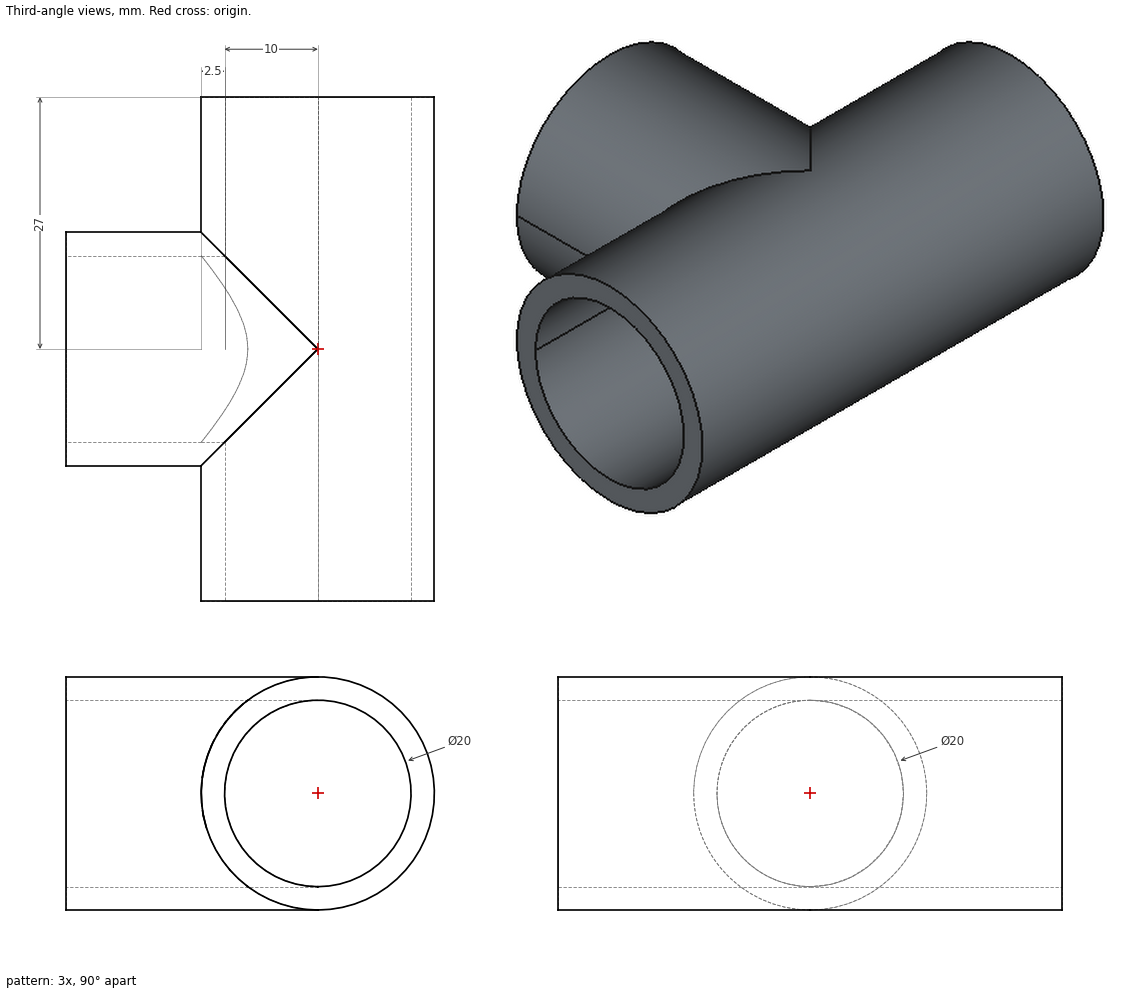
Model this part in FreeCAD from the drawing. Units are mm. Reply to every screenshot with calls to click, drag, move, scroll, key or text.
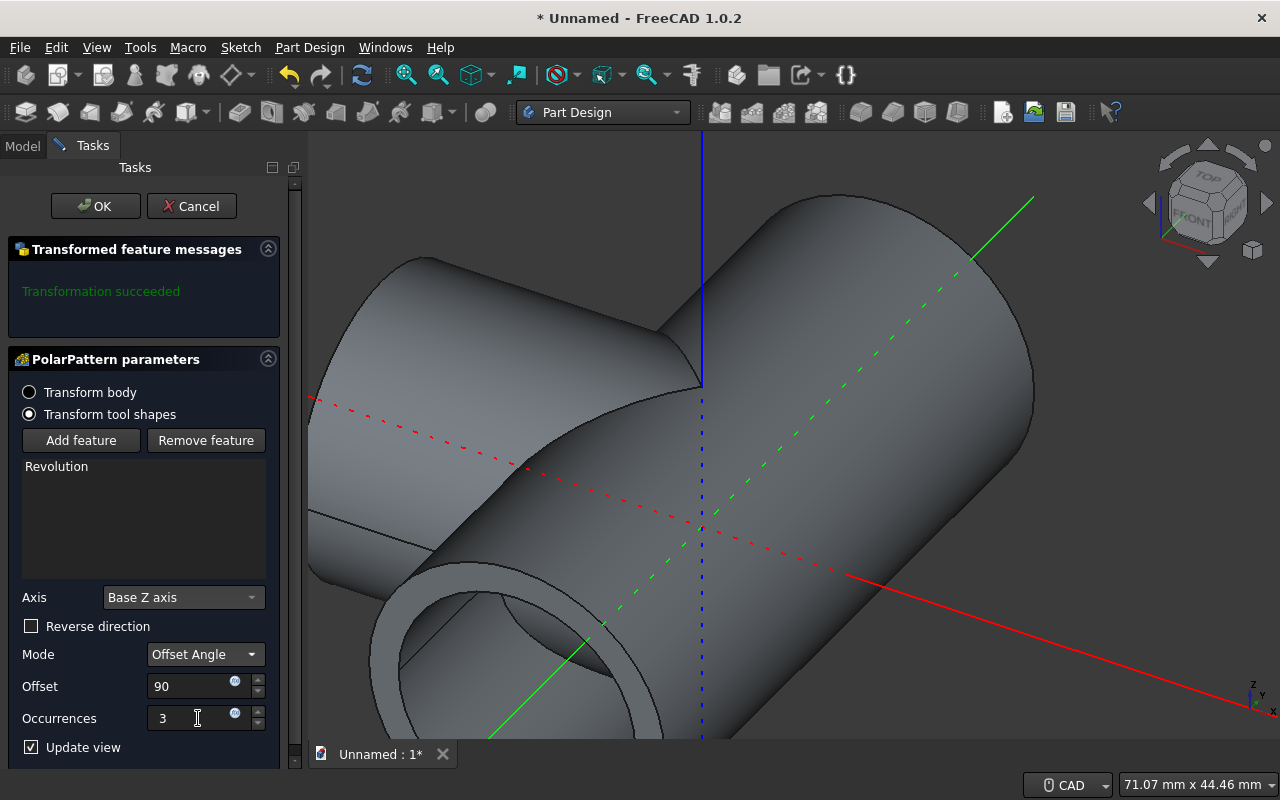
click(96, 206)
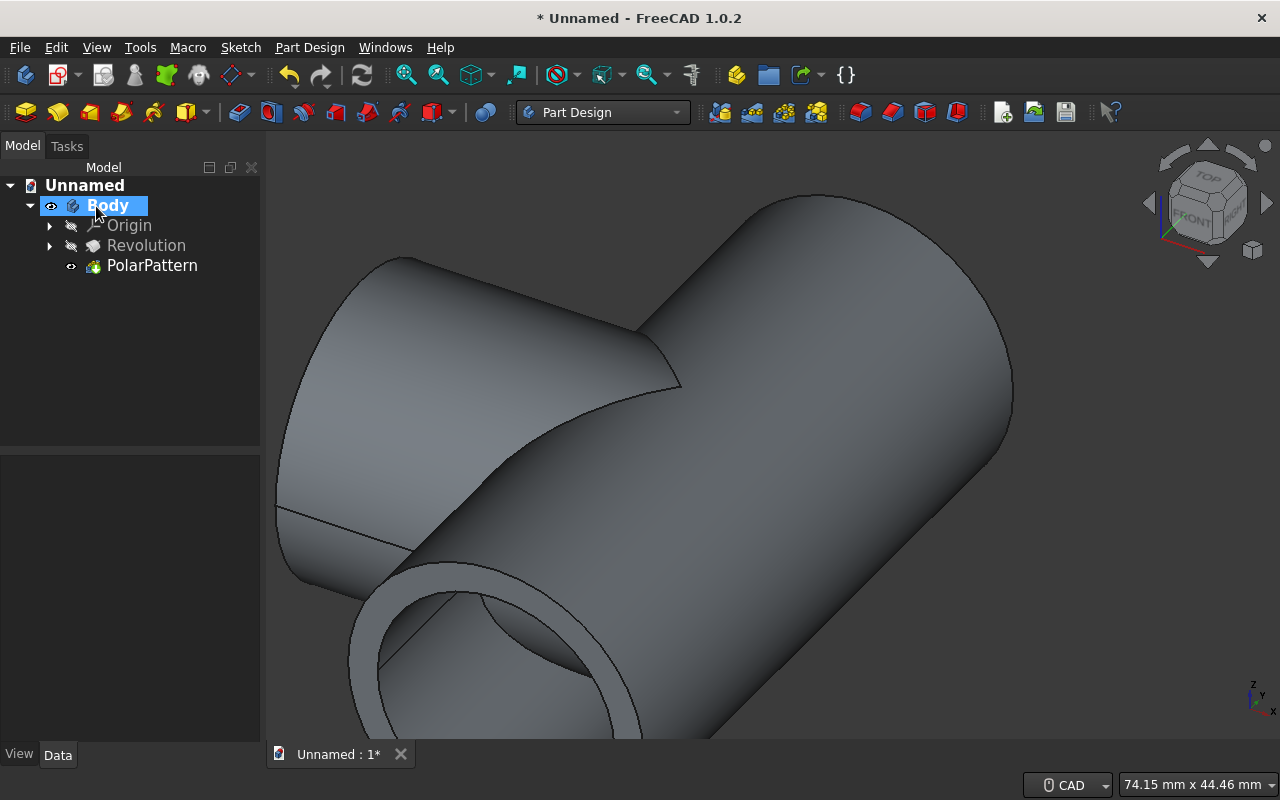
key(v)
key(f)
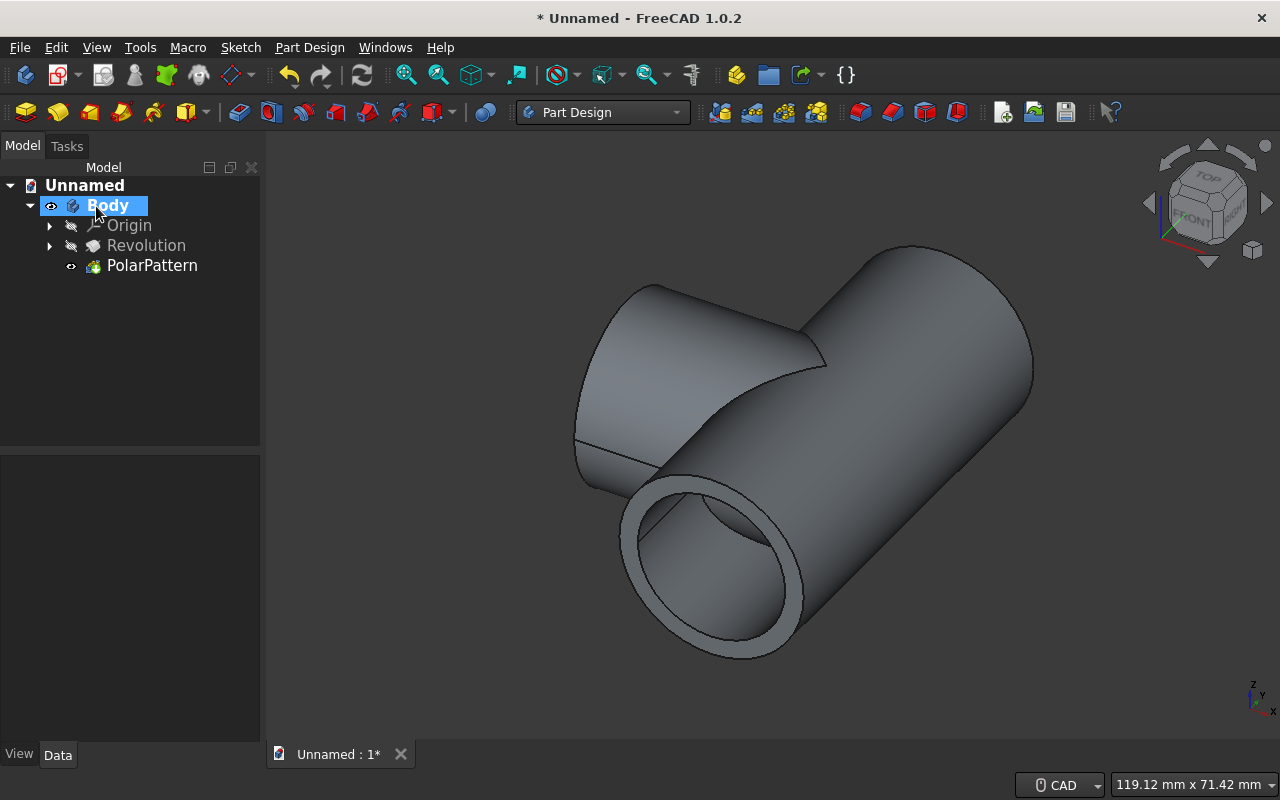
click(738, 649)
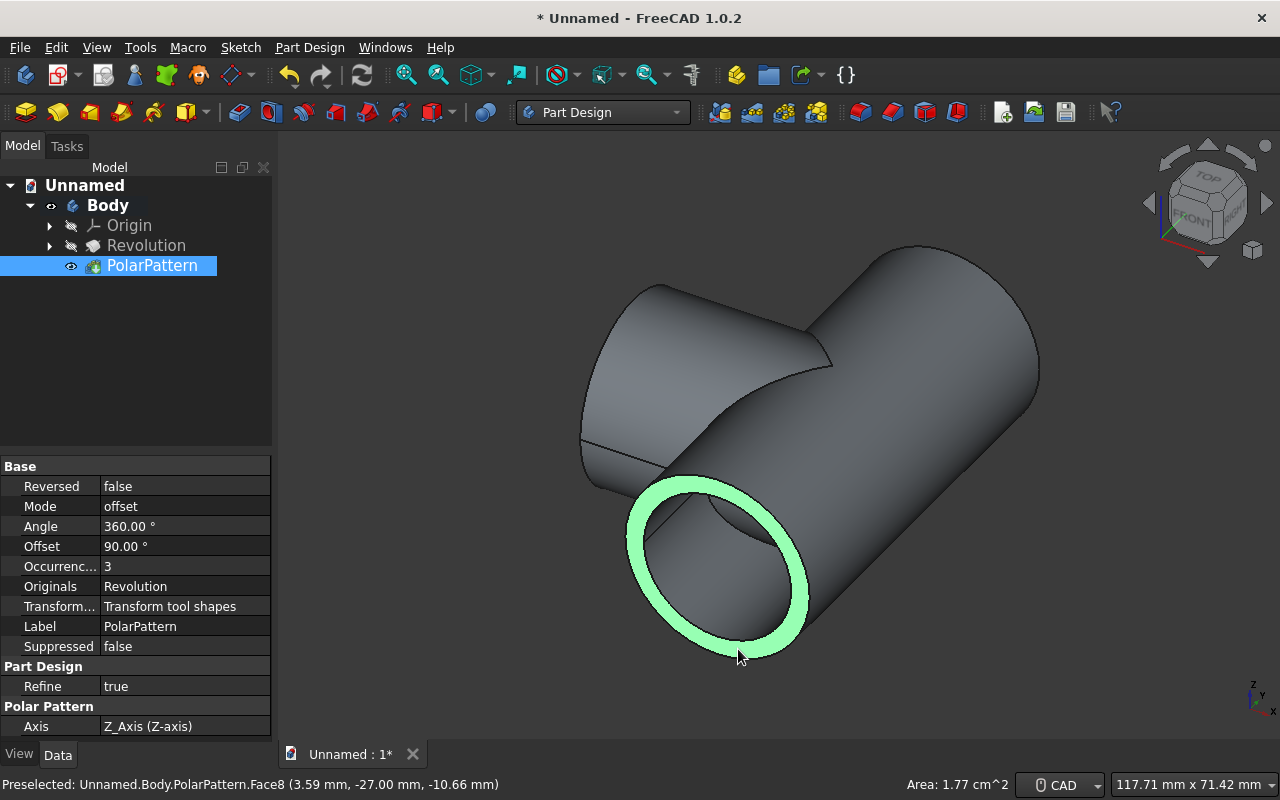
click(58, 76)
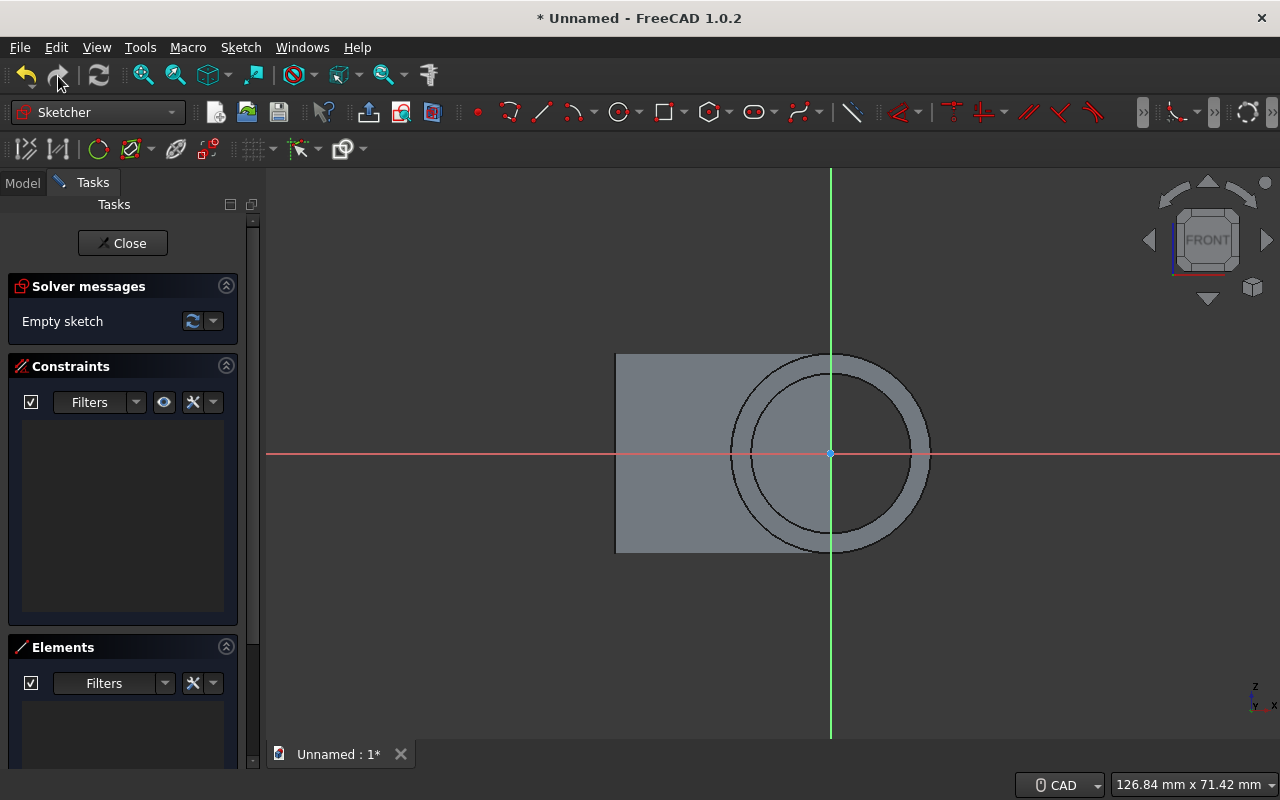
scroll(934, 454, up, 4)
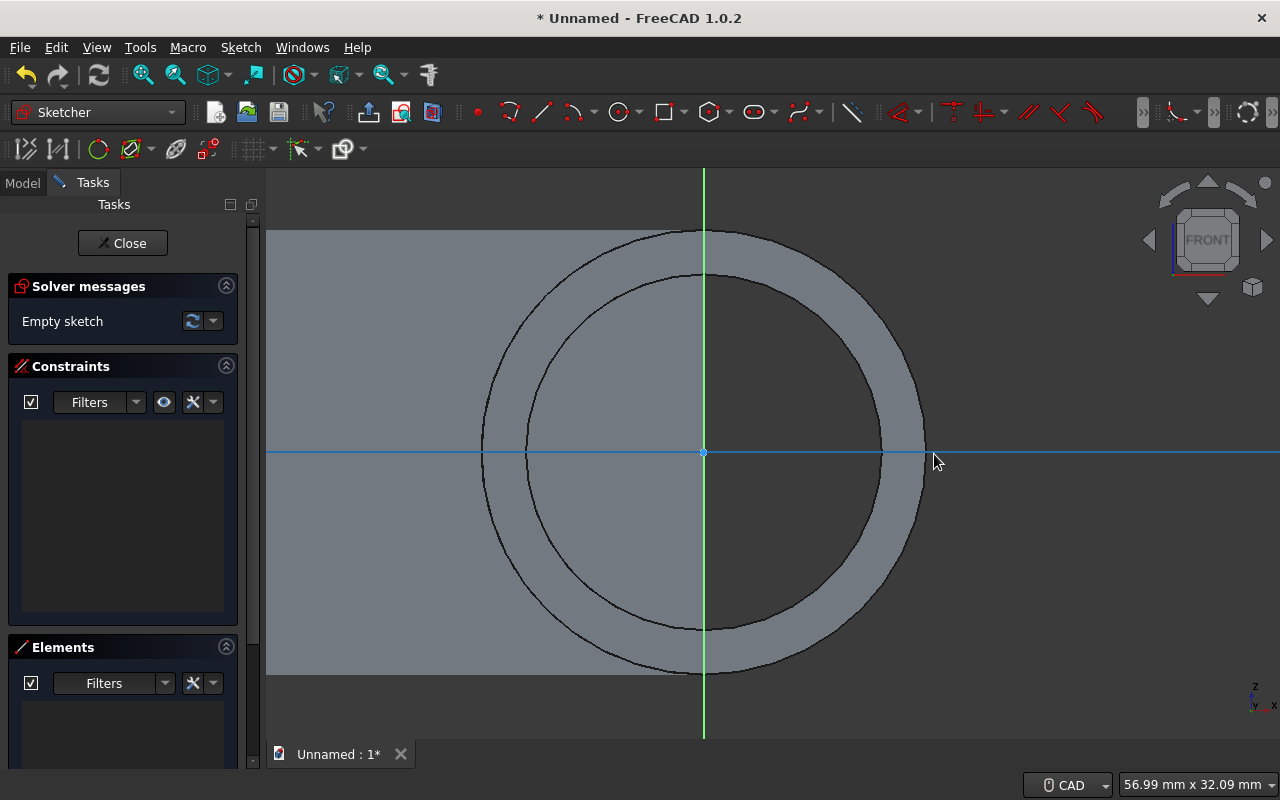
key(g)
key(c)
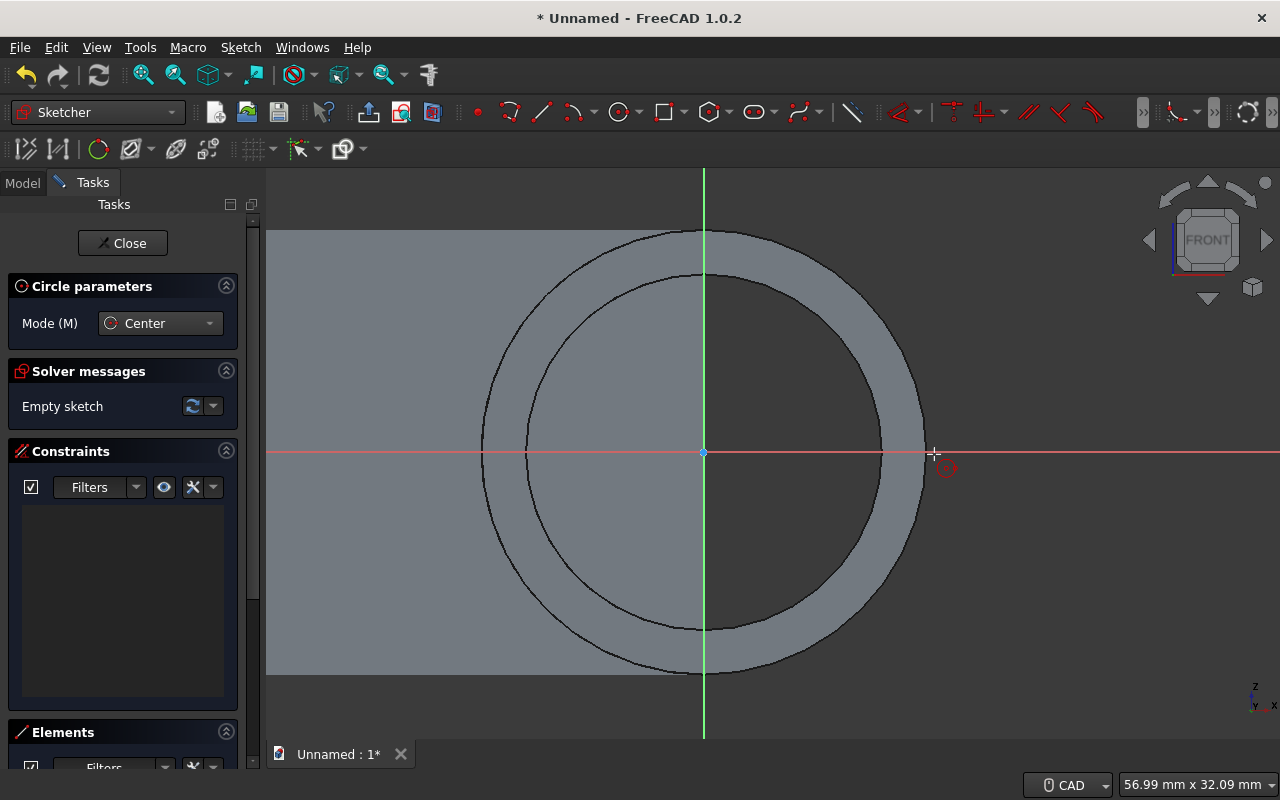
click(704, 452)
move(830, 326)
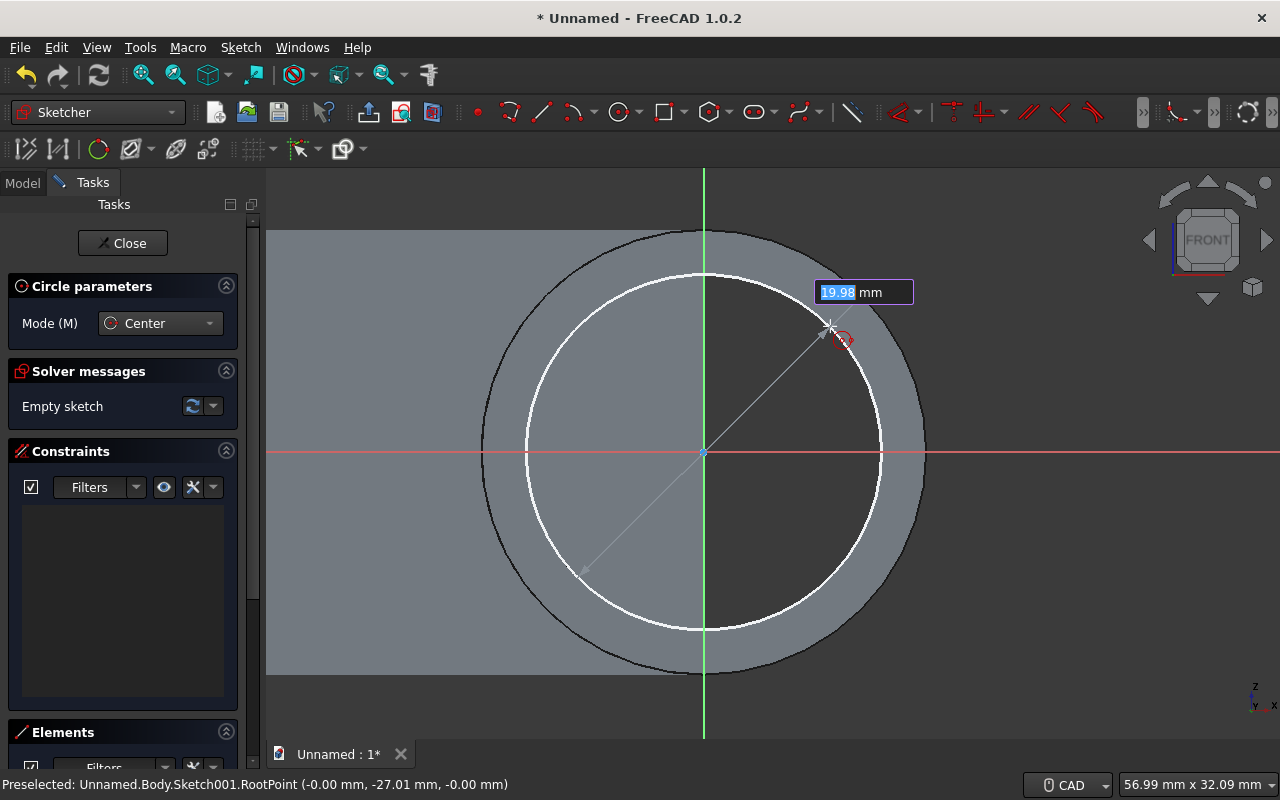
text(20)
key(Return)
key(Escape)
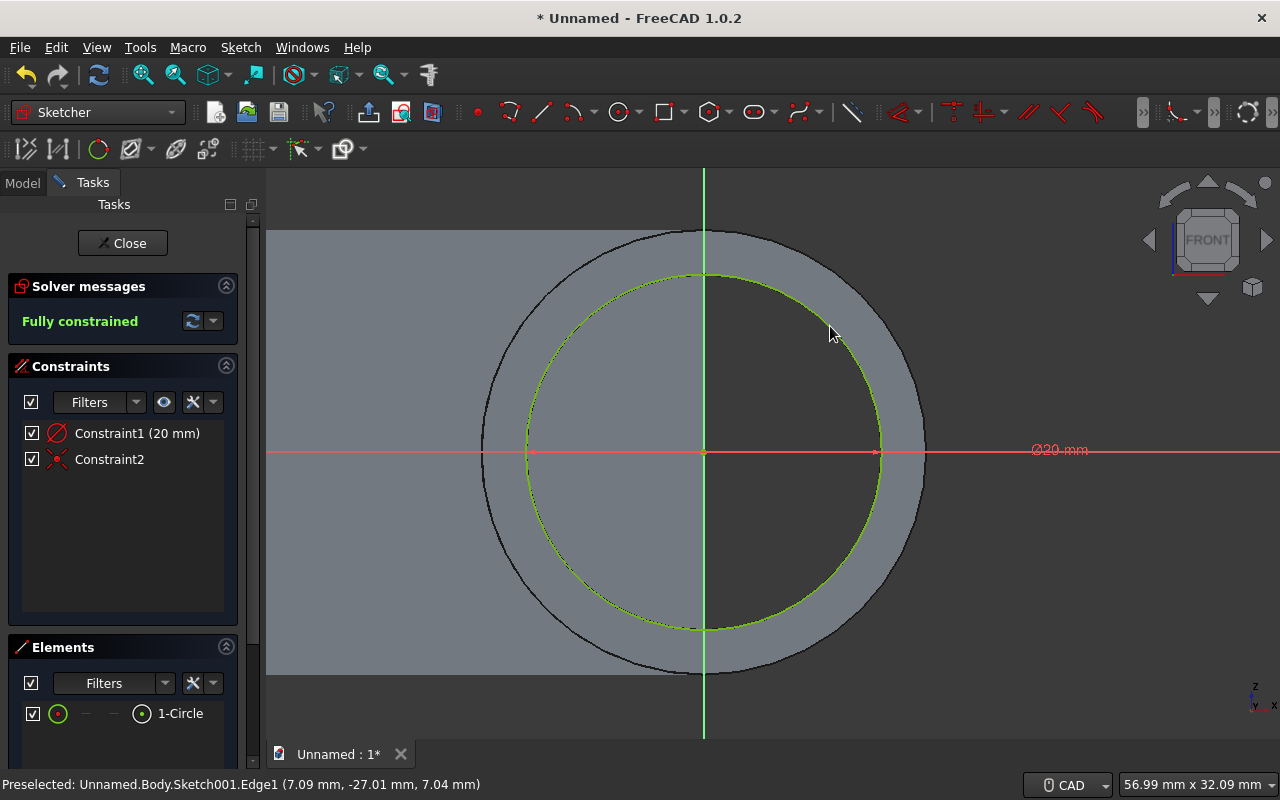
click(123, 243)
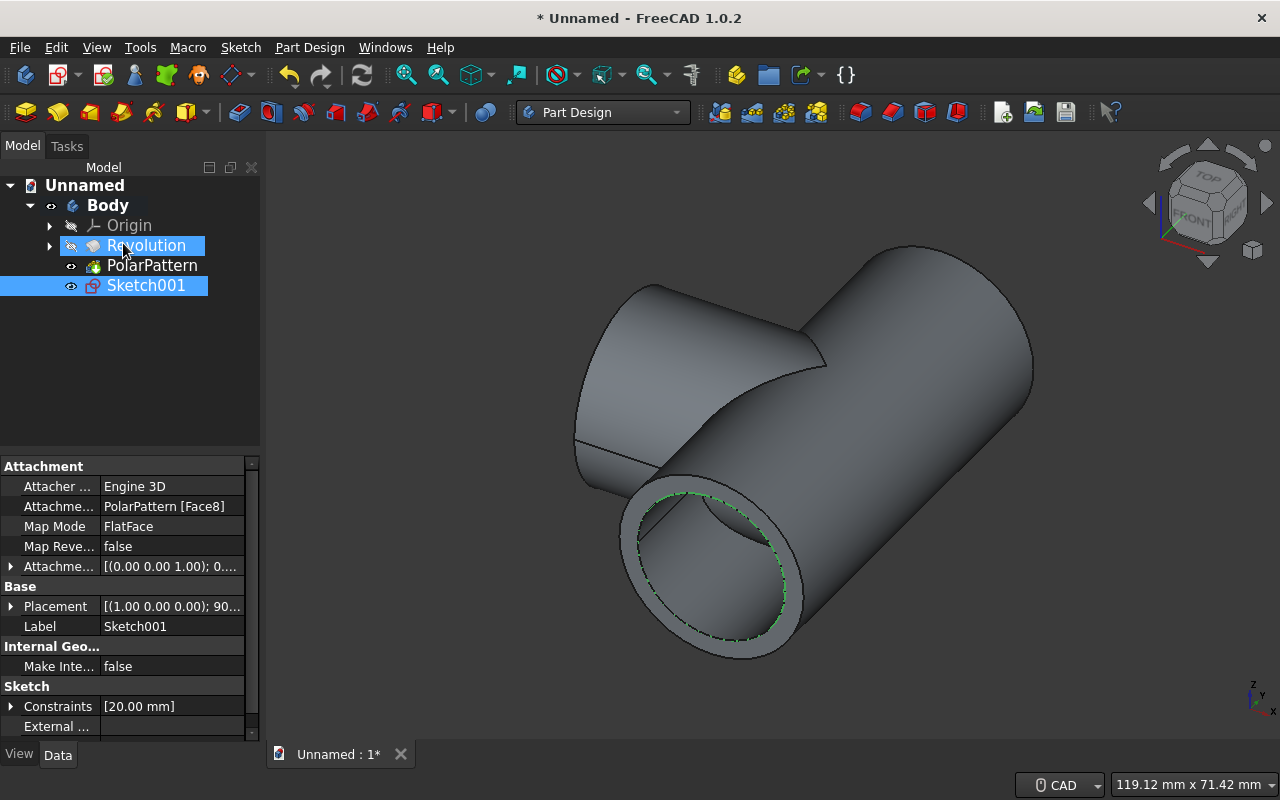
click(240, 112)